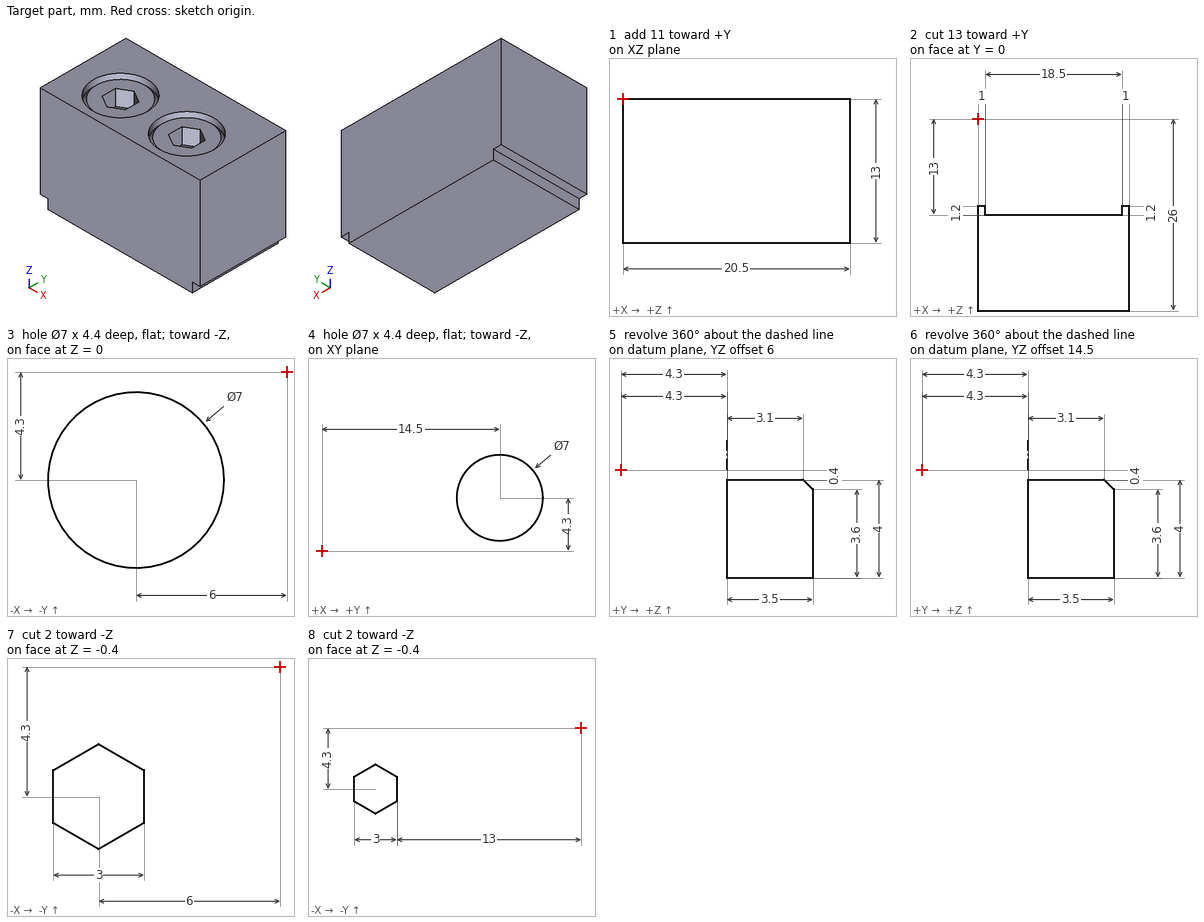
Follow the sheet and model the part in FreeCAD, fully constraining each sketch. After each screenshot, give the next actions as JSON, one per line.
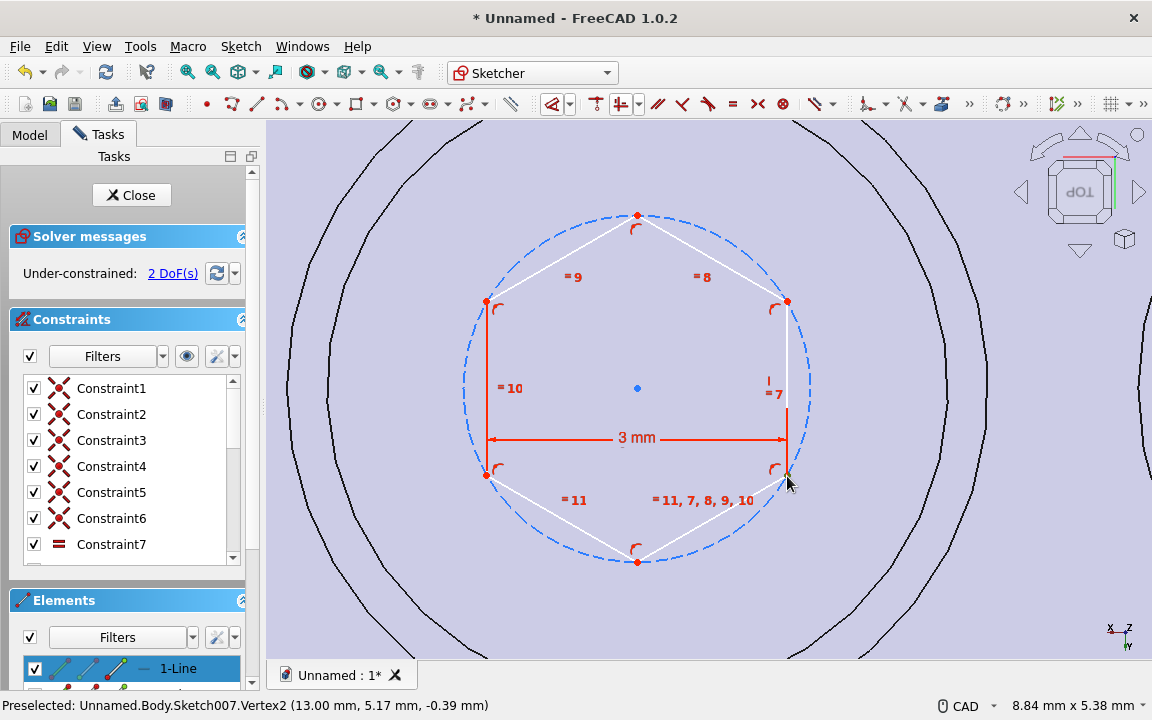
{"action": "left_click", "coordinate": [570, 104]}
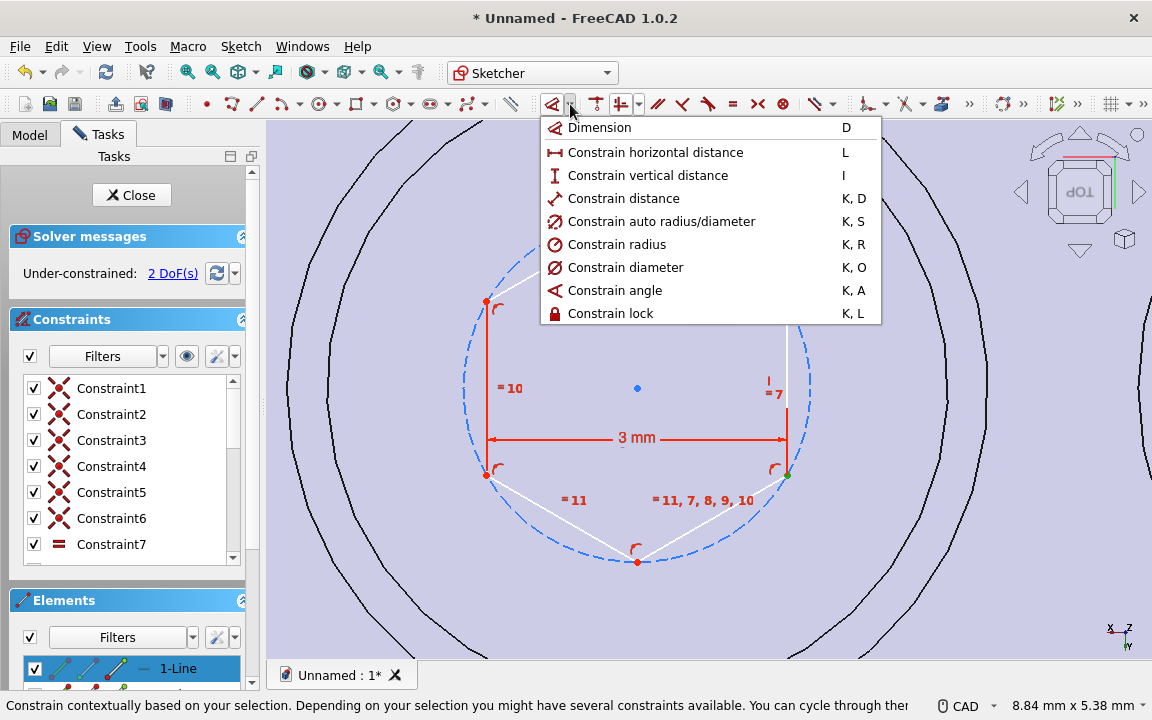
{"action": "left_click", "coordinate": [711, 152]}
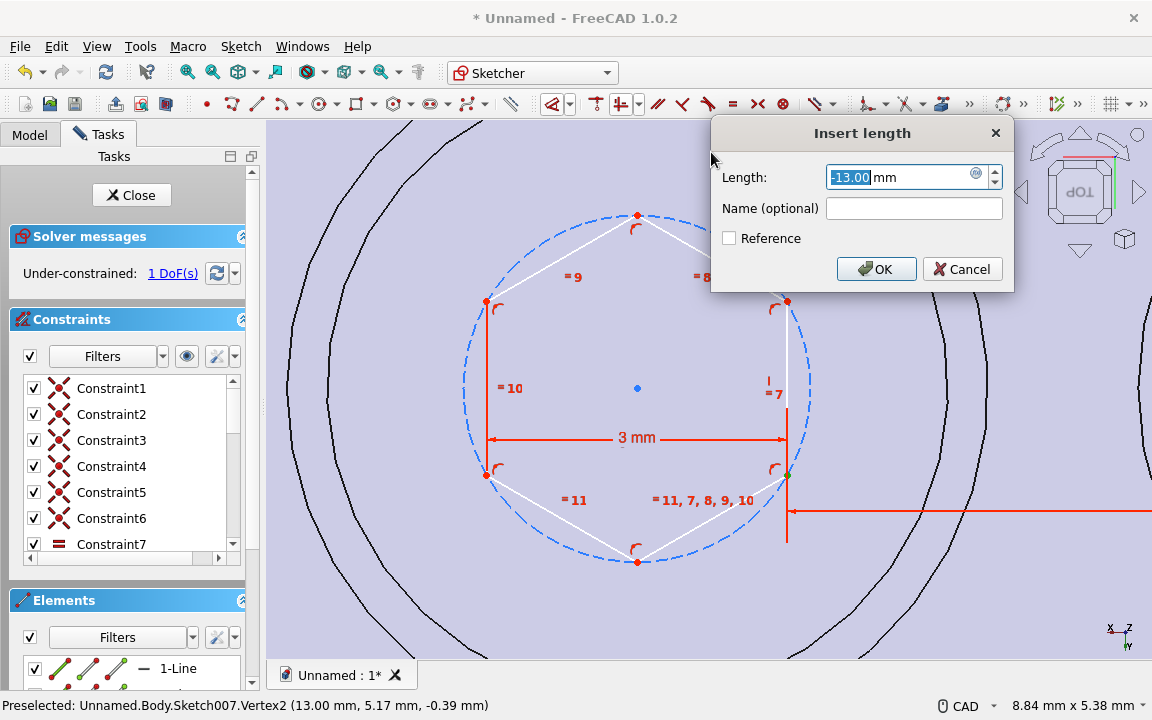
{"action": "type", "text": "-13"}
{"action": "key", "text": "Return"}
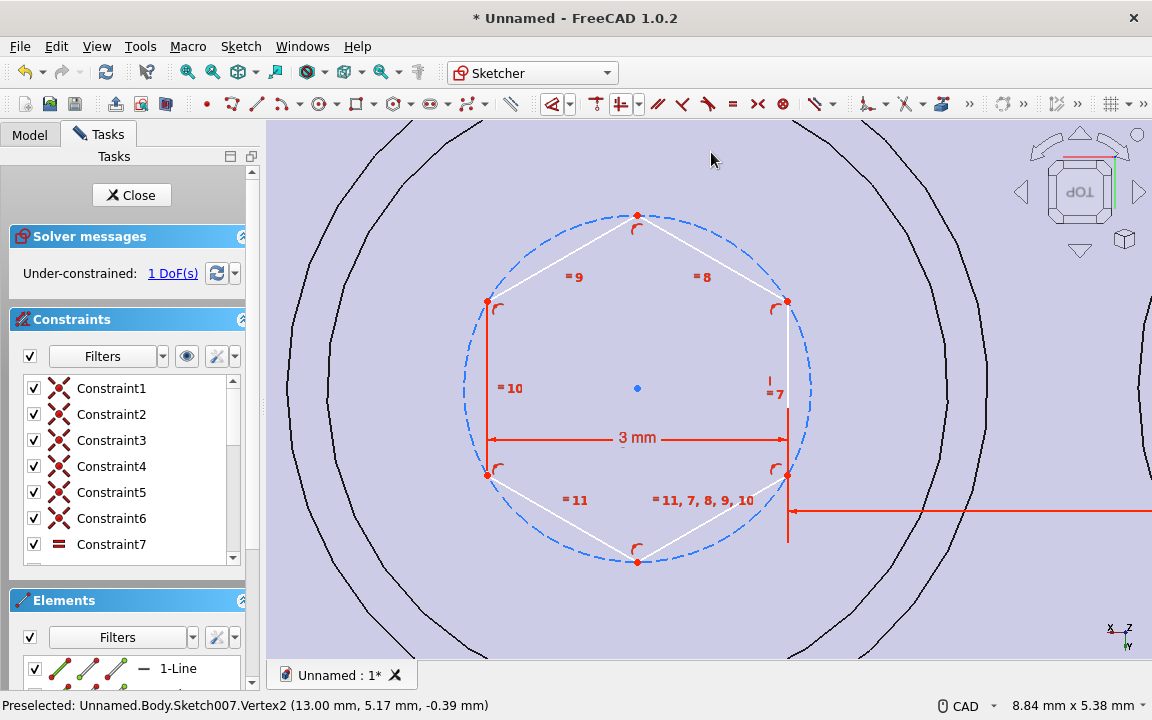
{"action": "left_click", "coordinate": [637, 389]}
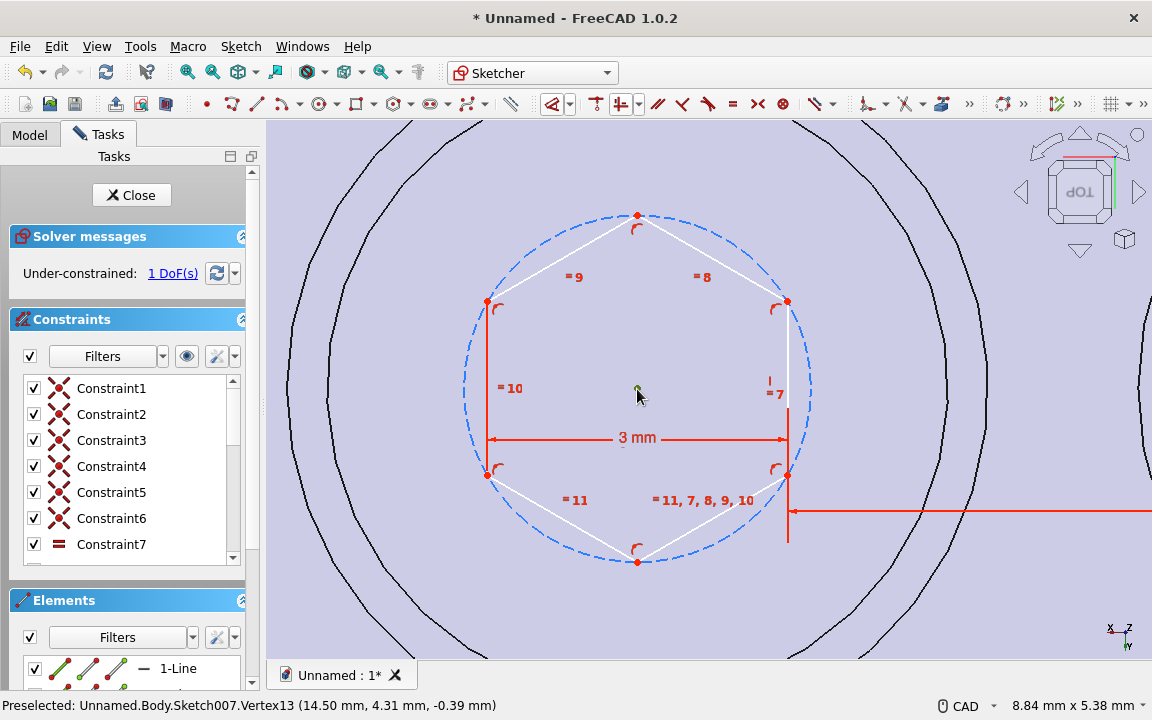
{"action": "key", "text": "i"}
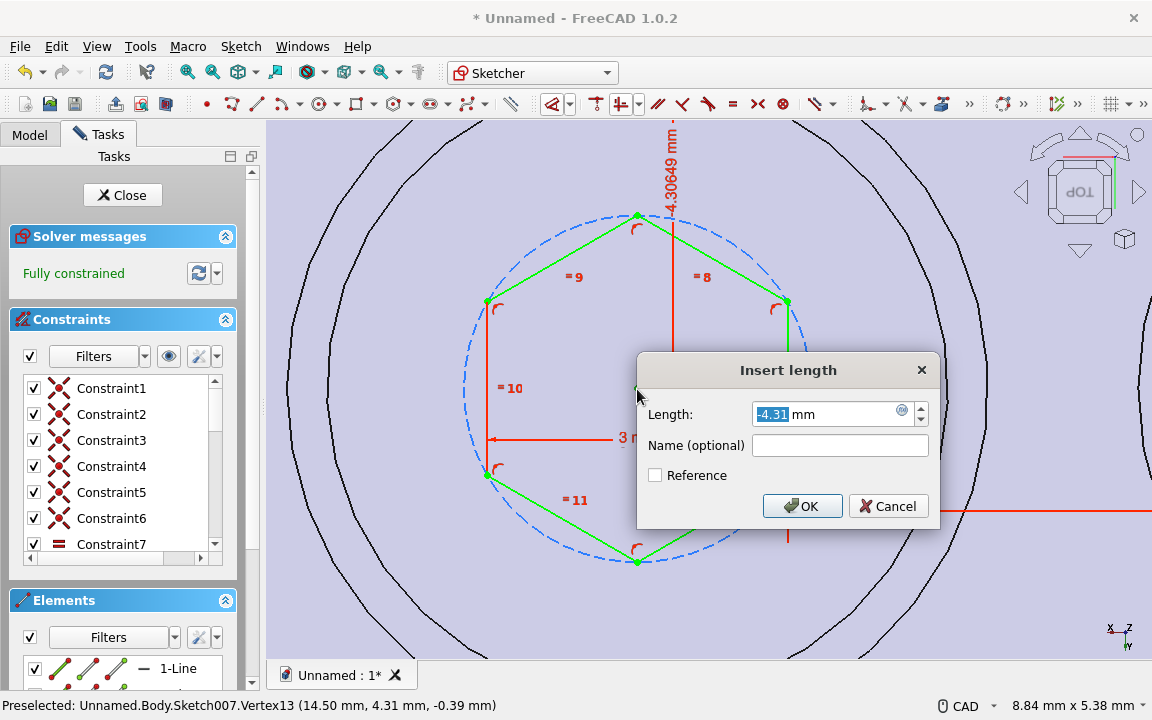
{"action": "type", "text": "-4.3"}
{"action": "key", "text": "Return"}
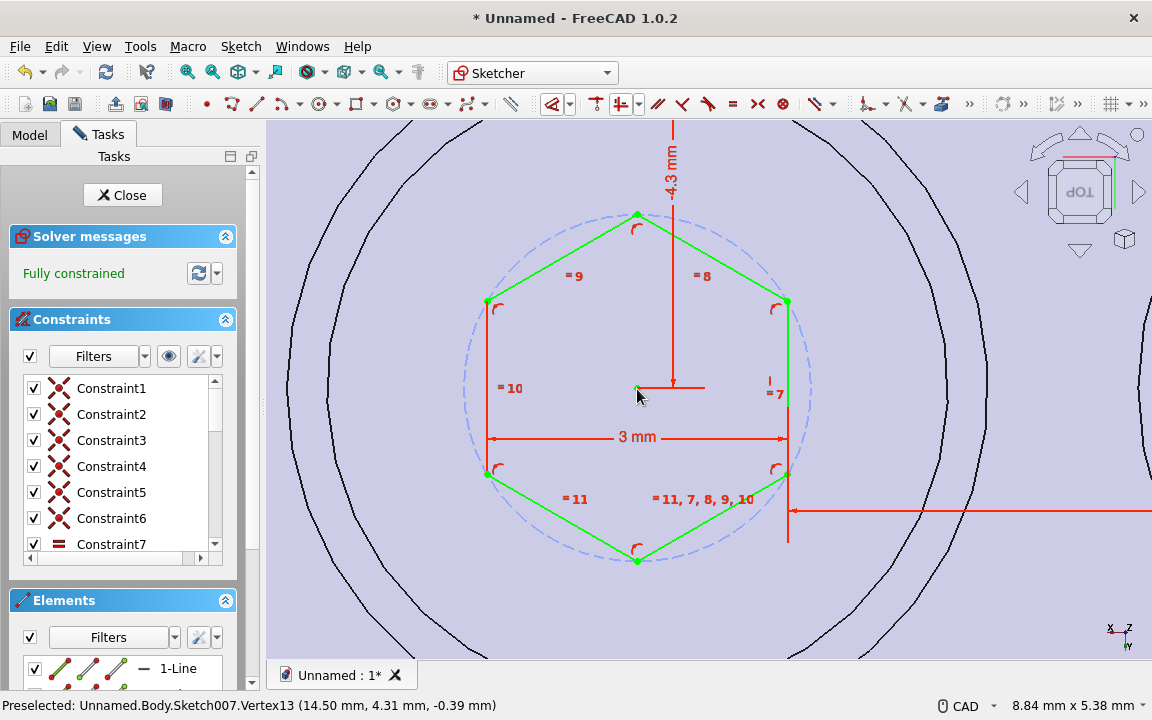
{"action": "left_click", "coordinate": [123, 195]}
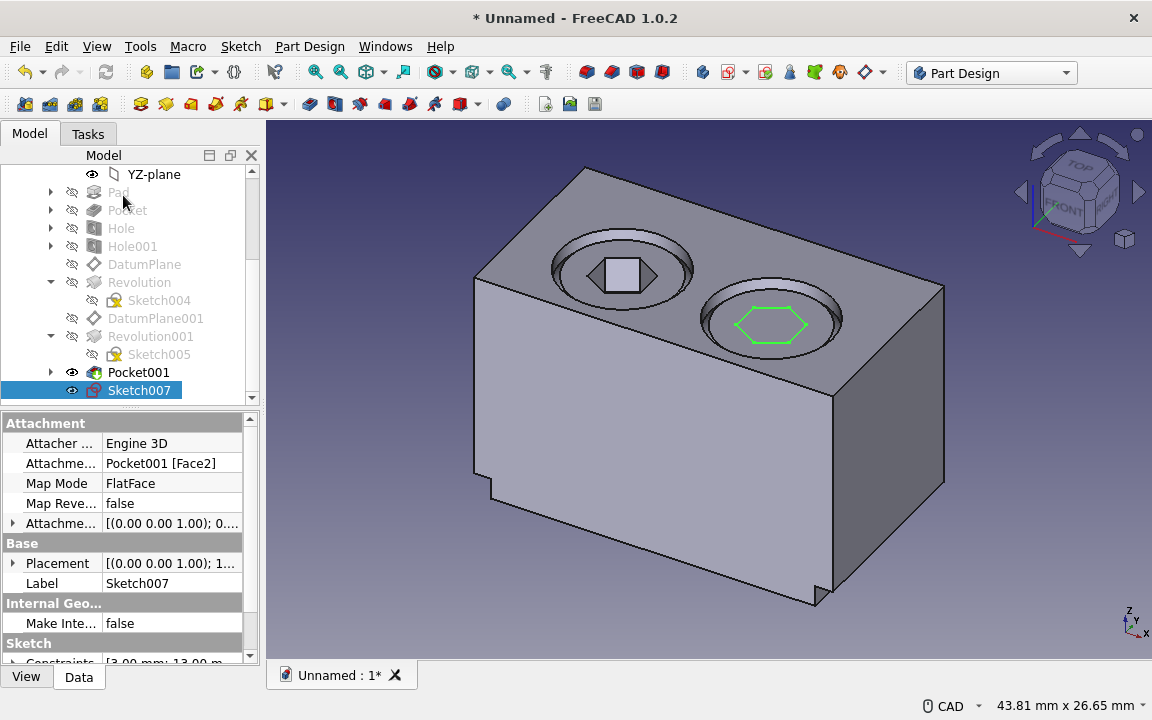
{"action": "left_click", "coordinate": [310, 104]}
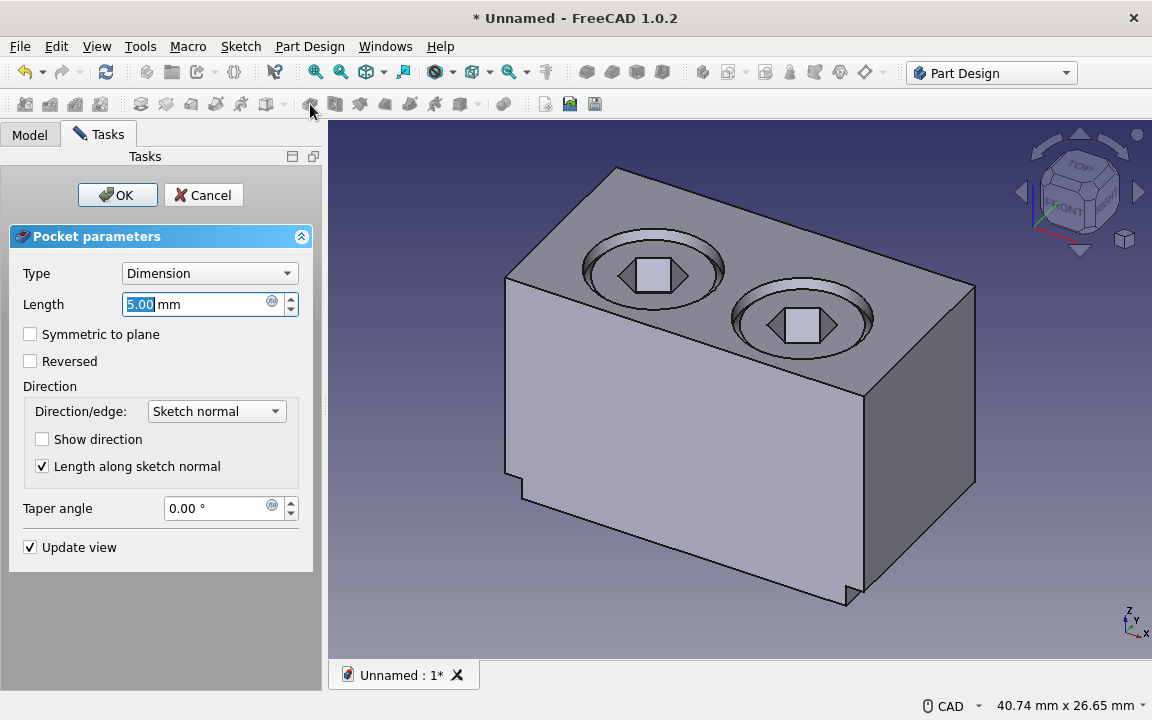
{"action": "type", "text": "2"}
{"action": "key", "text": "Tab"}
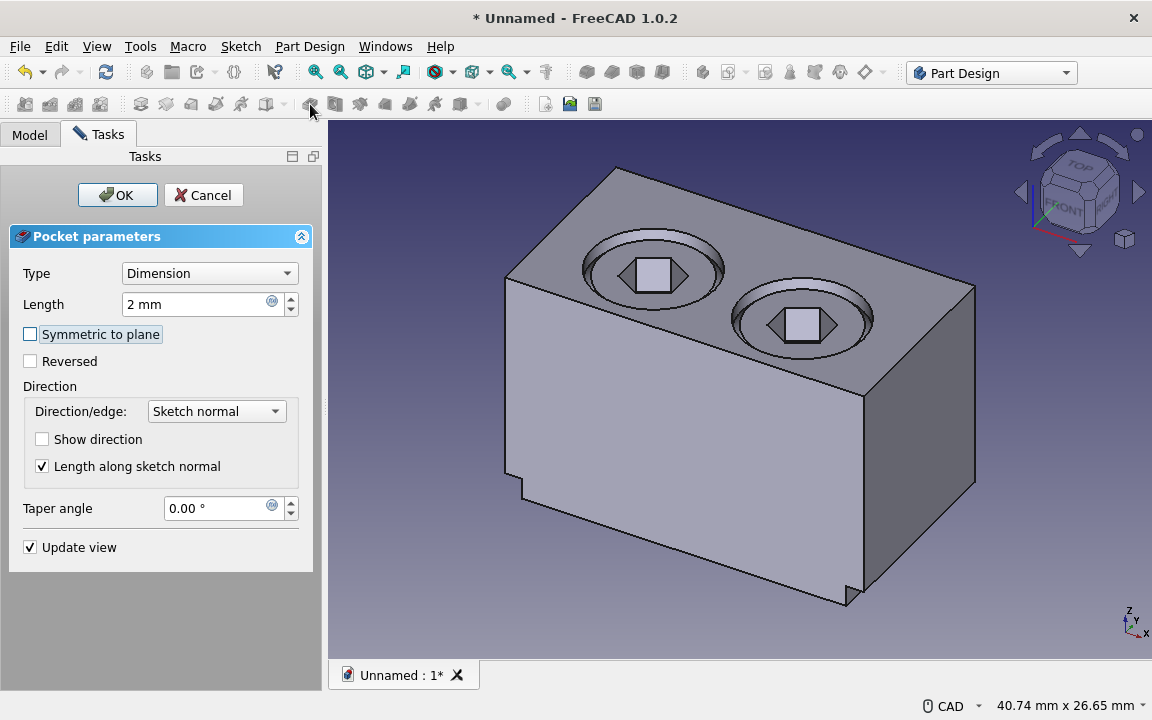
{"action": "left_click", "coordinate": [118, 195]}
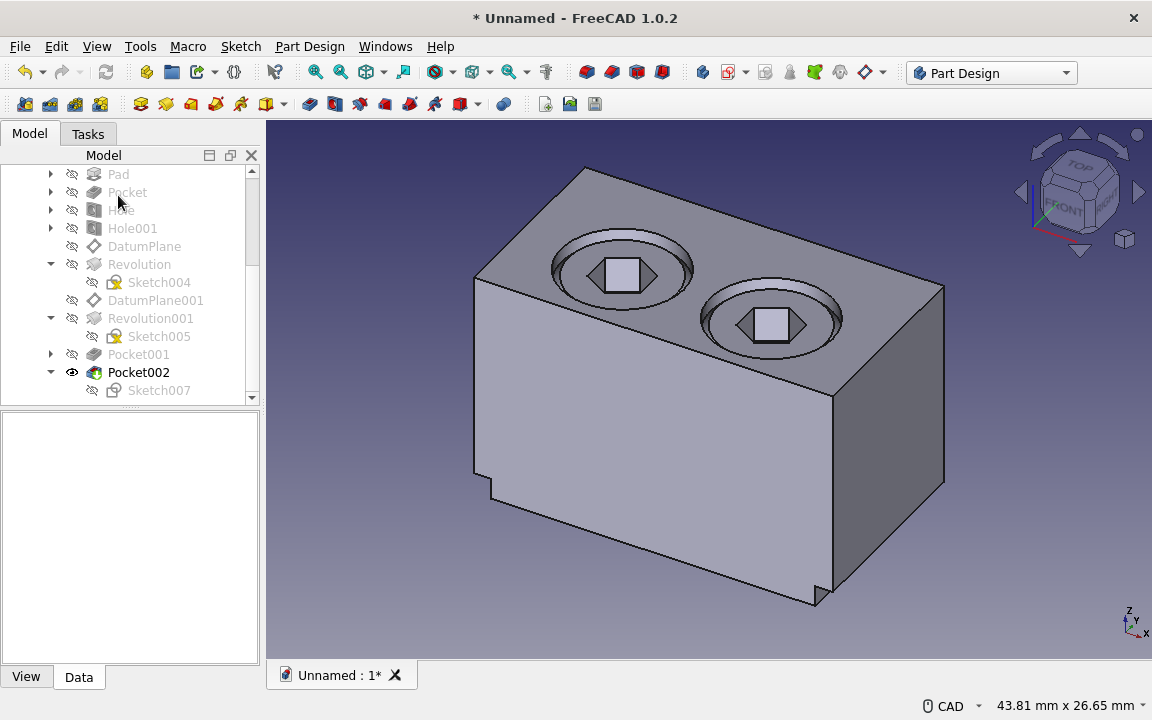
{"action": "key", "text": "0"}